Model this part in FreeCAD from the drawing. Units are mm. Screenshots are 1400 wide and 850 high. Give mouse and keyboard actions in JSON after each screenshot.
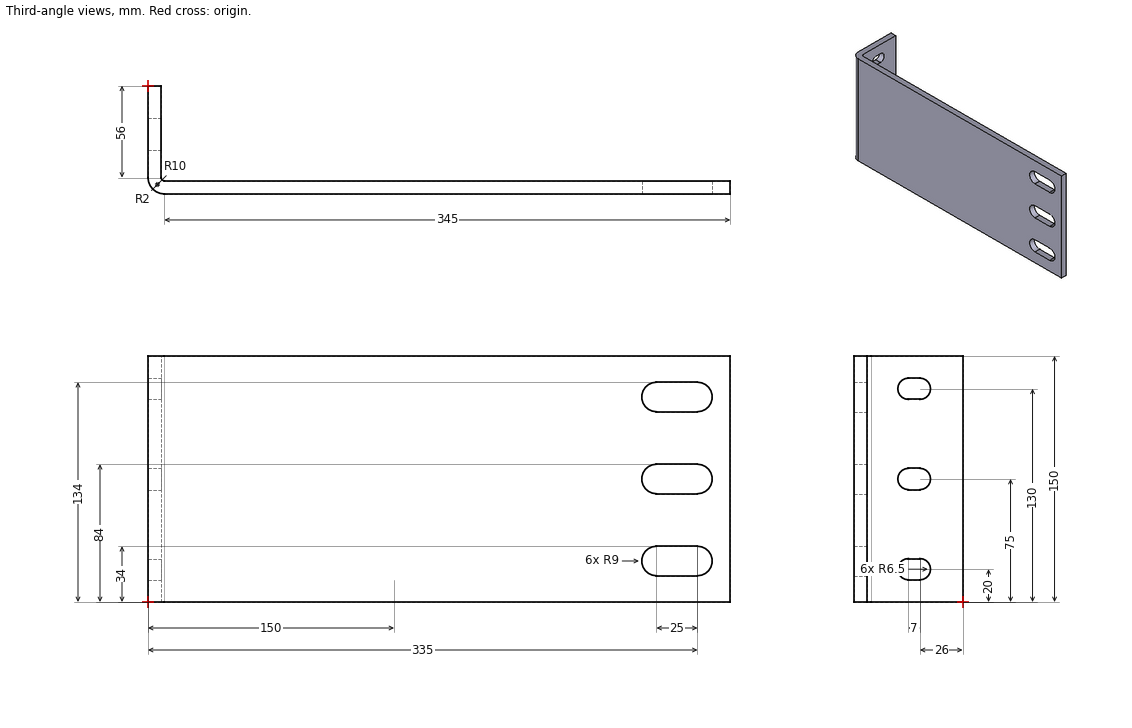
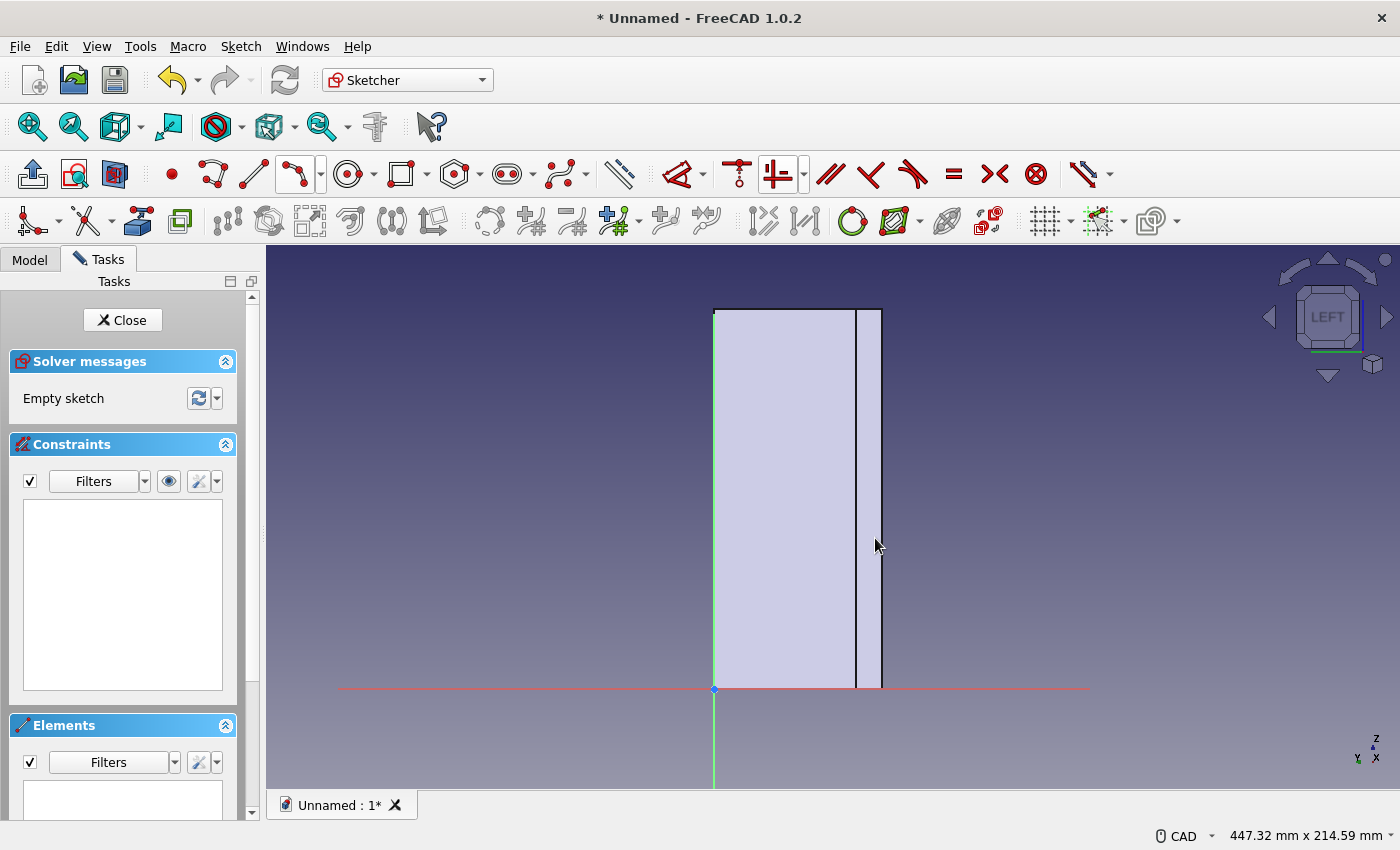
{"action": "left_click", "coordinate": [506, 174]}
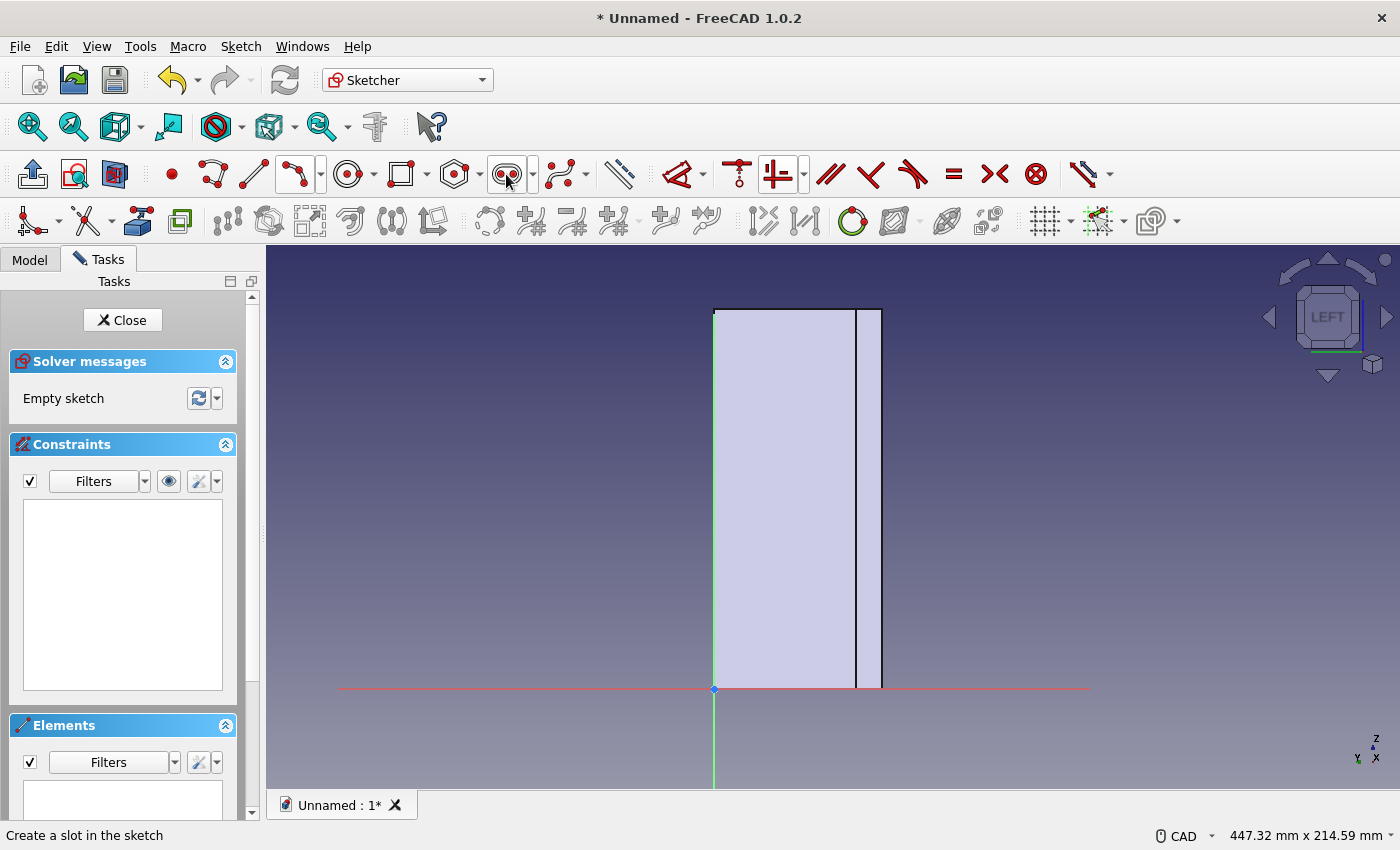
{"action": "scroll", "coordinate": [780, 639], "scroll_direction": "up", "scroll_amount": 2}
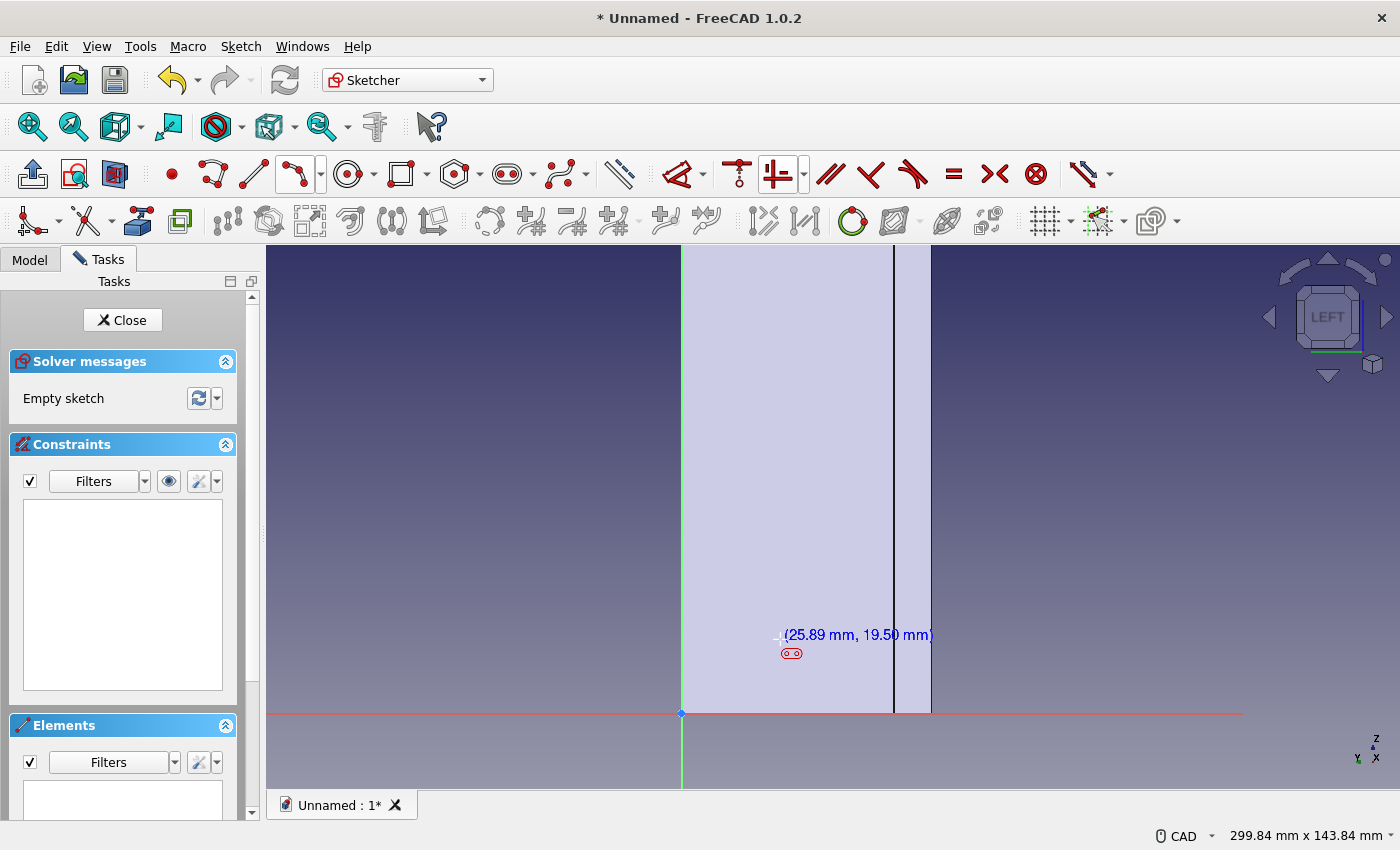
{"action": "left_click", "coordinate": [780, 638]}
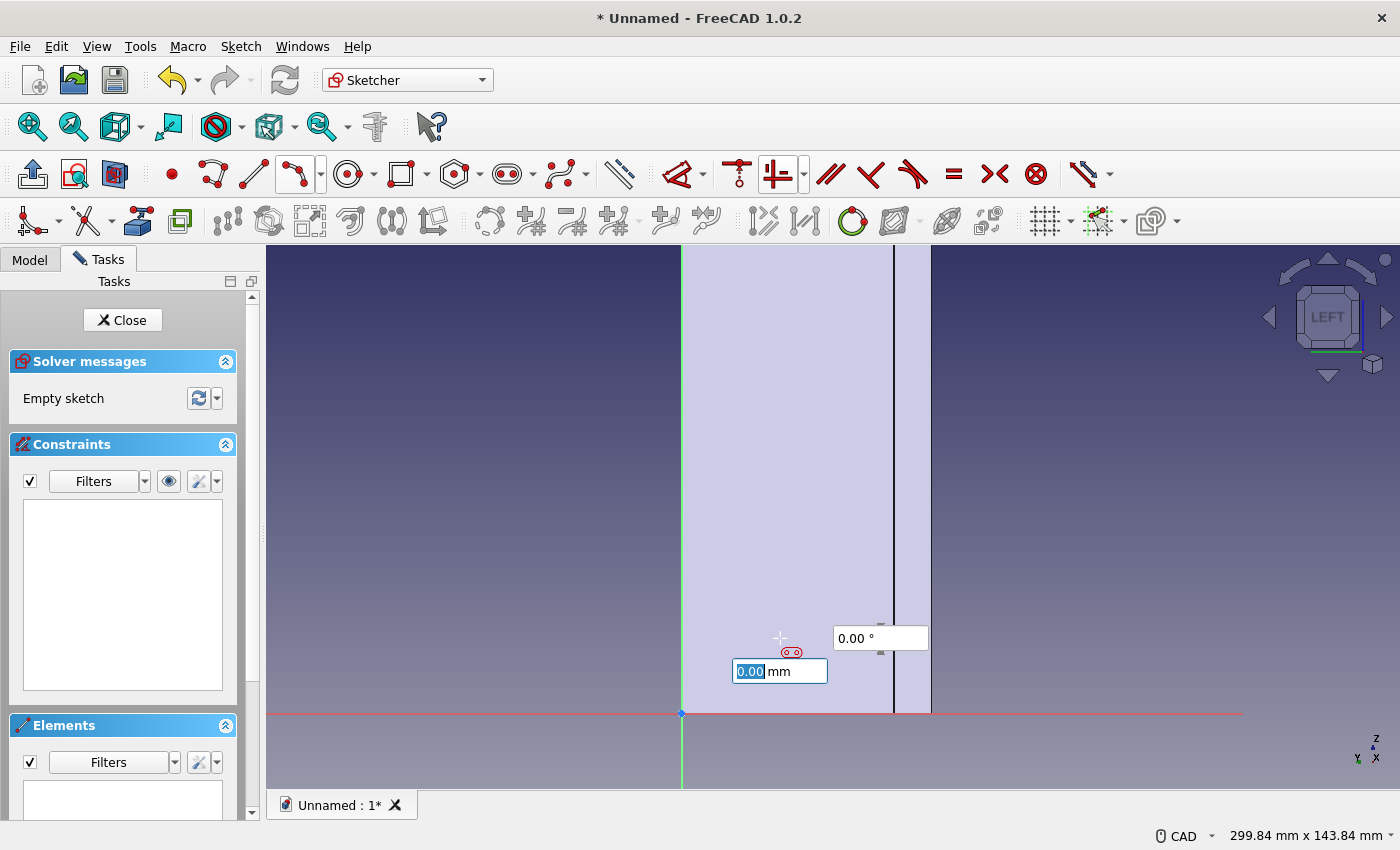
{"action": "left_click", "coordinate": [807, 638]}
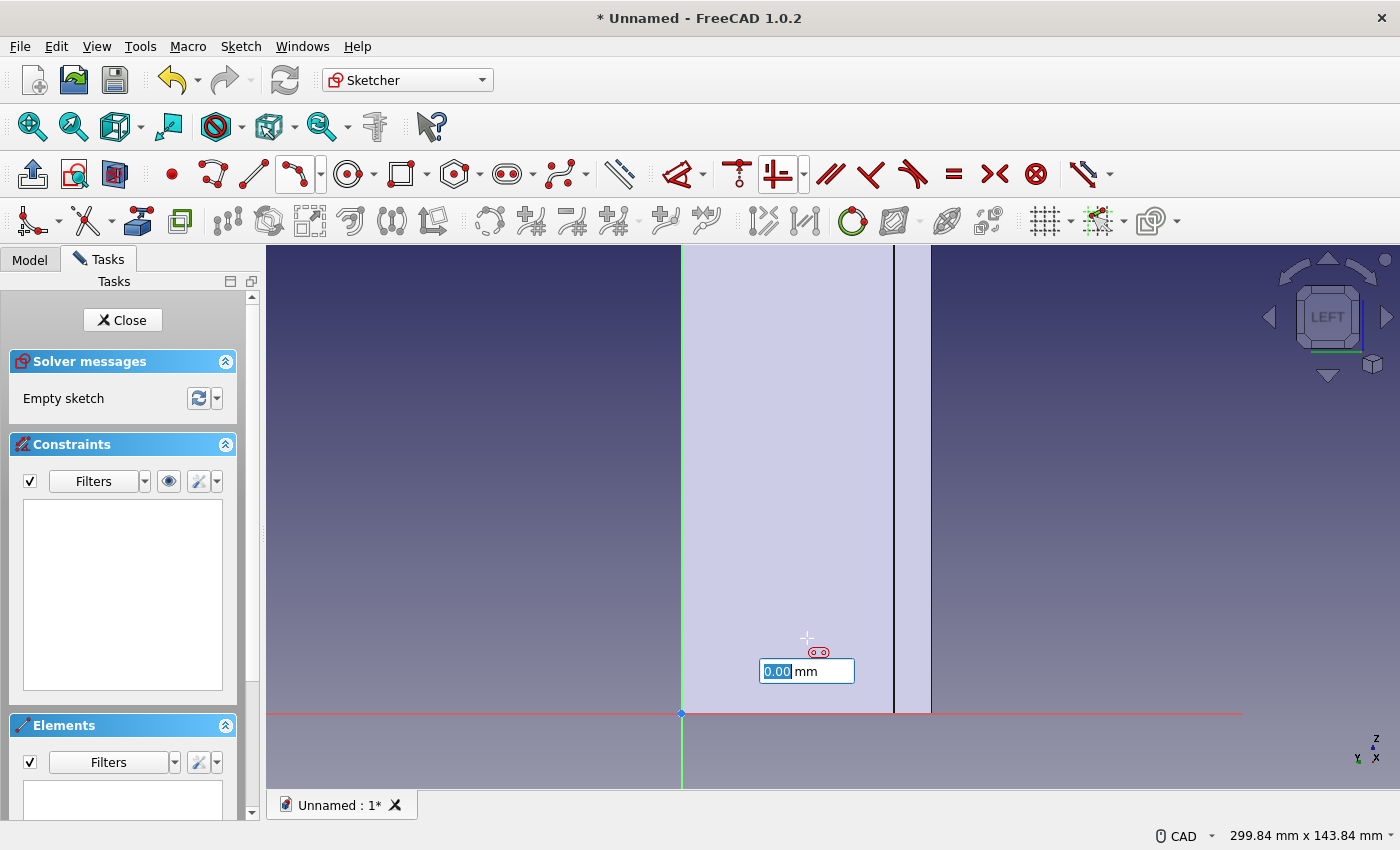
{"action": "left_click", "coordinate": [793, 614]}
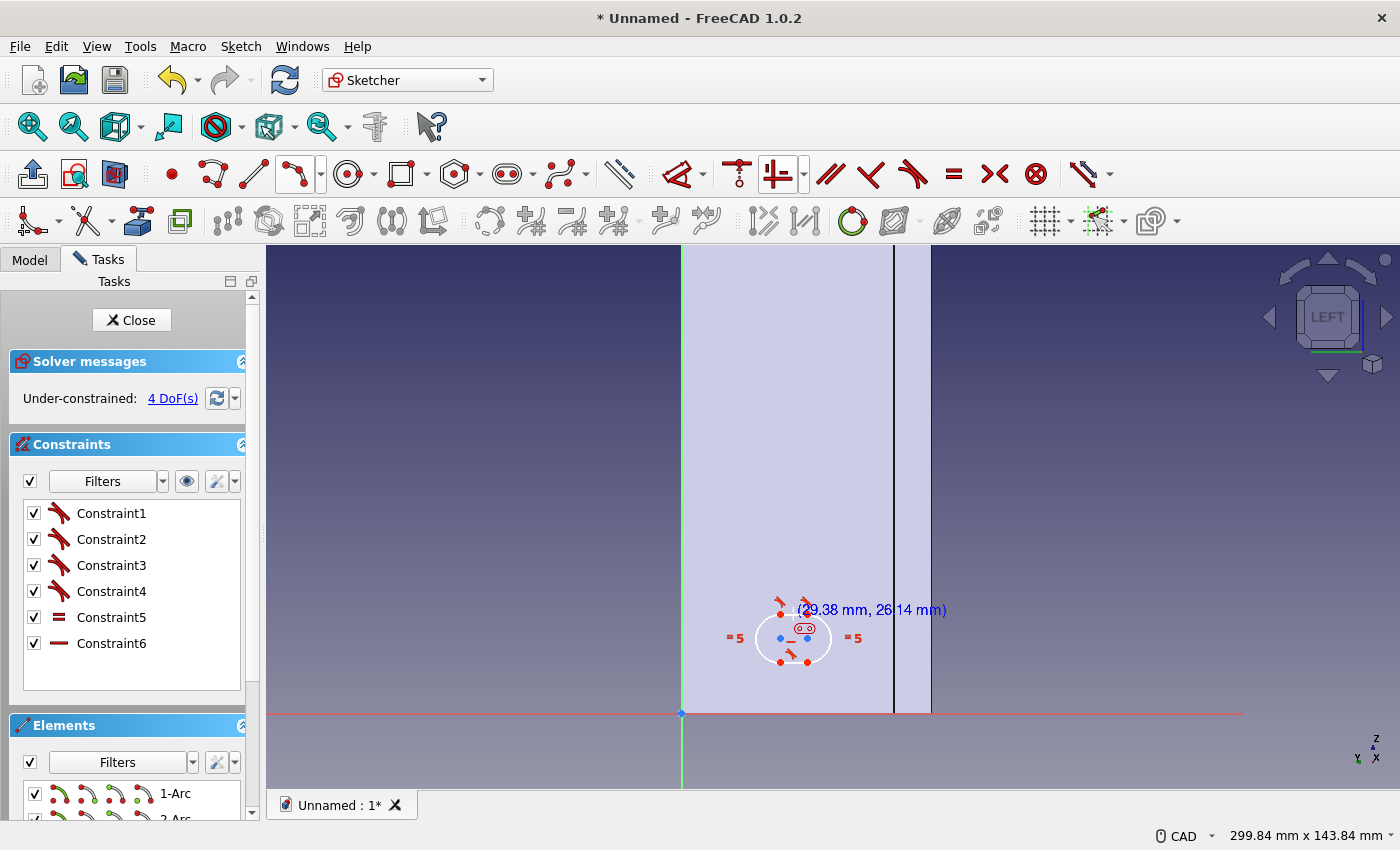
{"action": "left_click", "coordinate": [780, 430]}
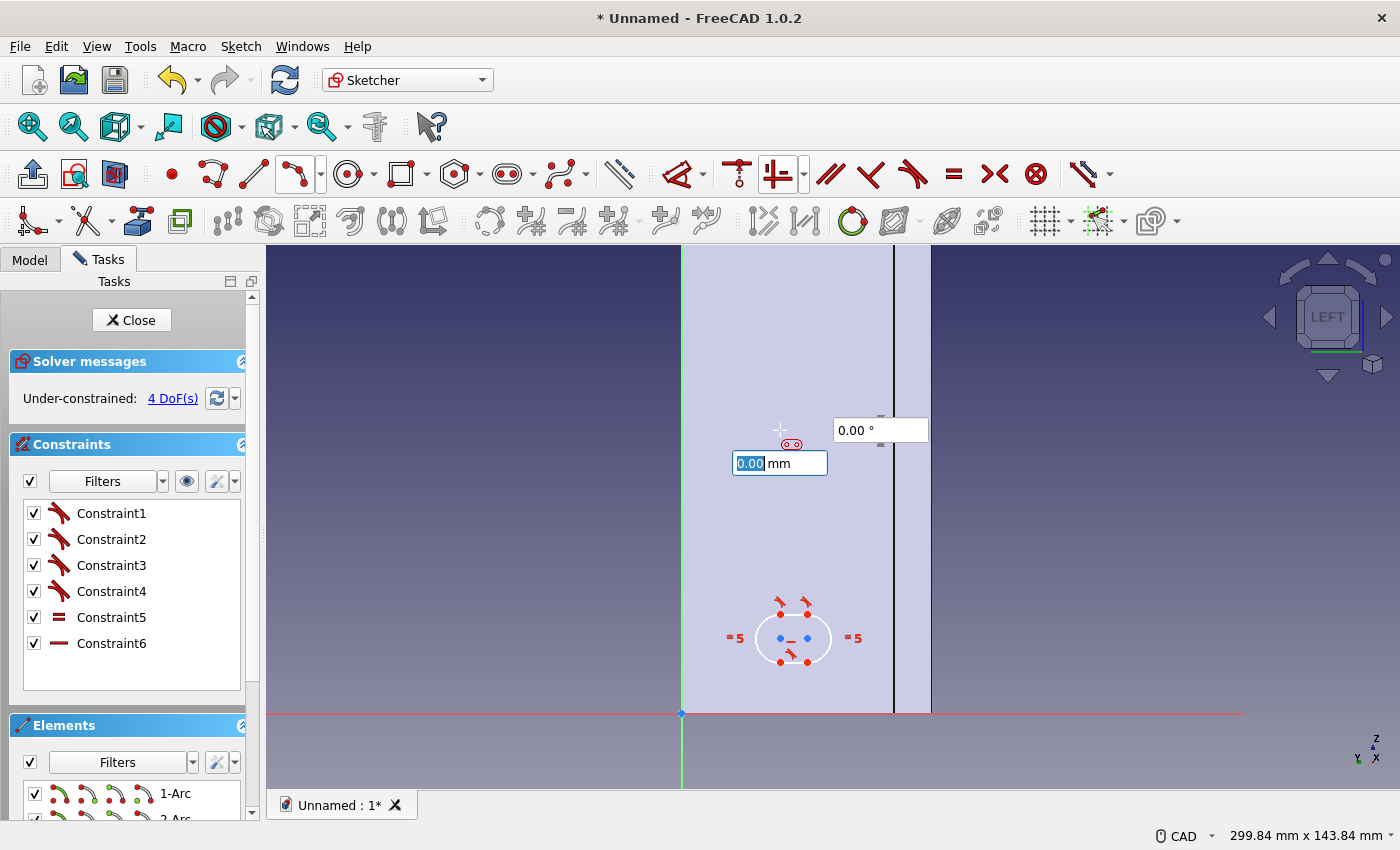
{"action": "left_click", "coordinate": [807, 430]}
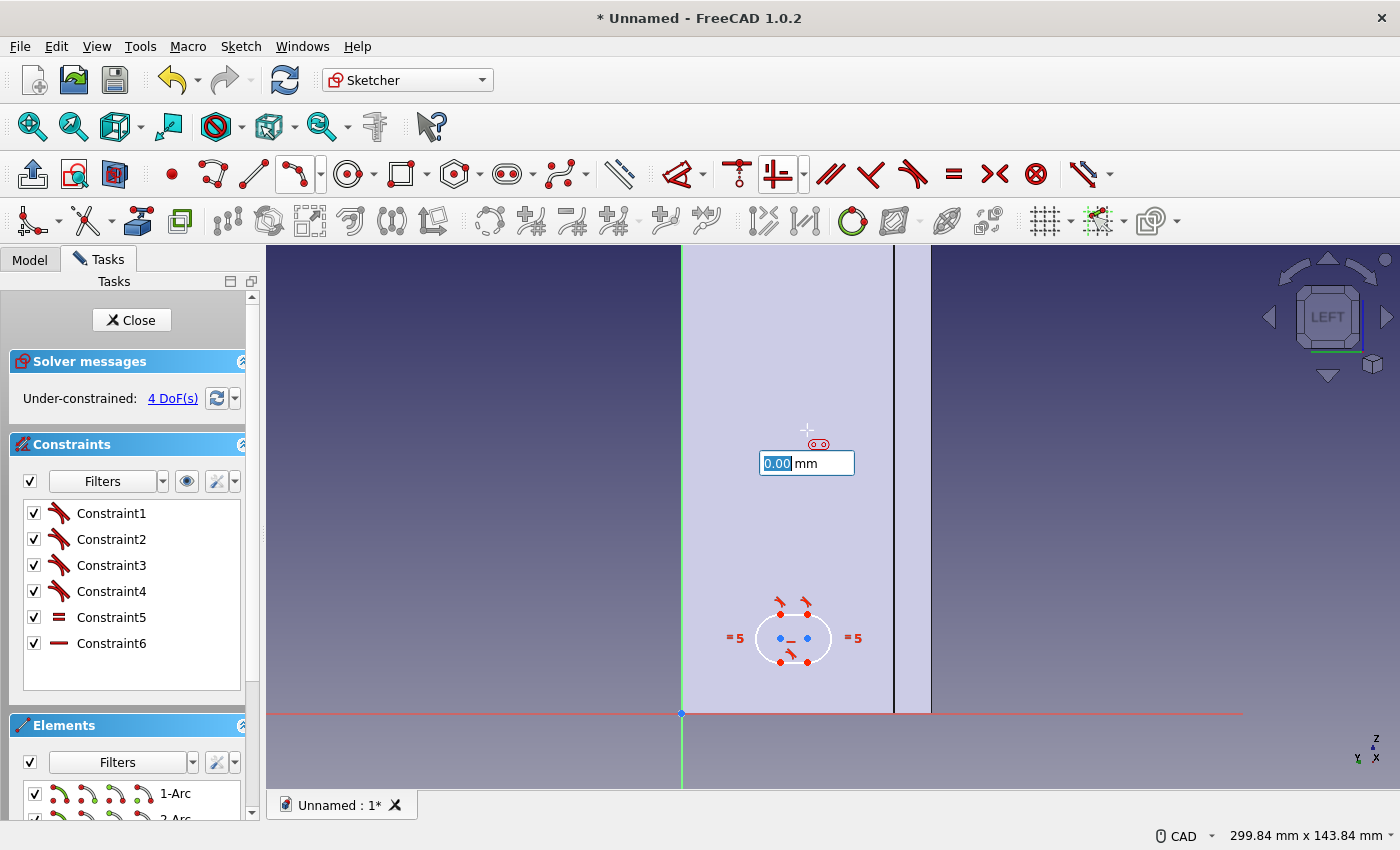
{"action": "left_click", "coordinate": [793, 406]}